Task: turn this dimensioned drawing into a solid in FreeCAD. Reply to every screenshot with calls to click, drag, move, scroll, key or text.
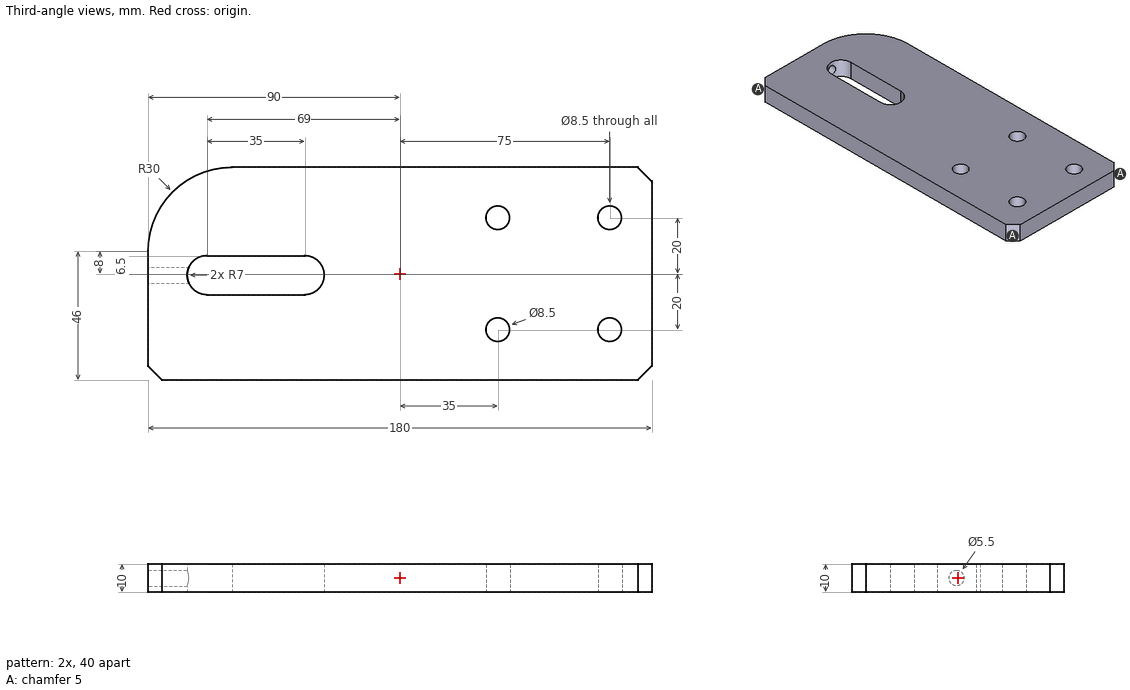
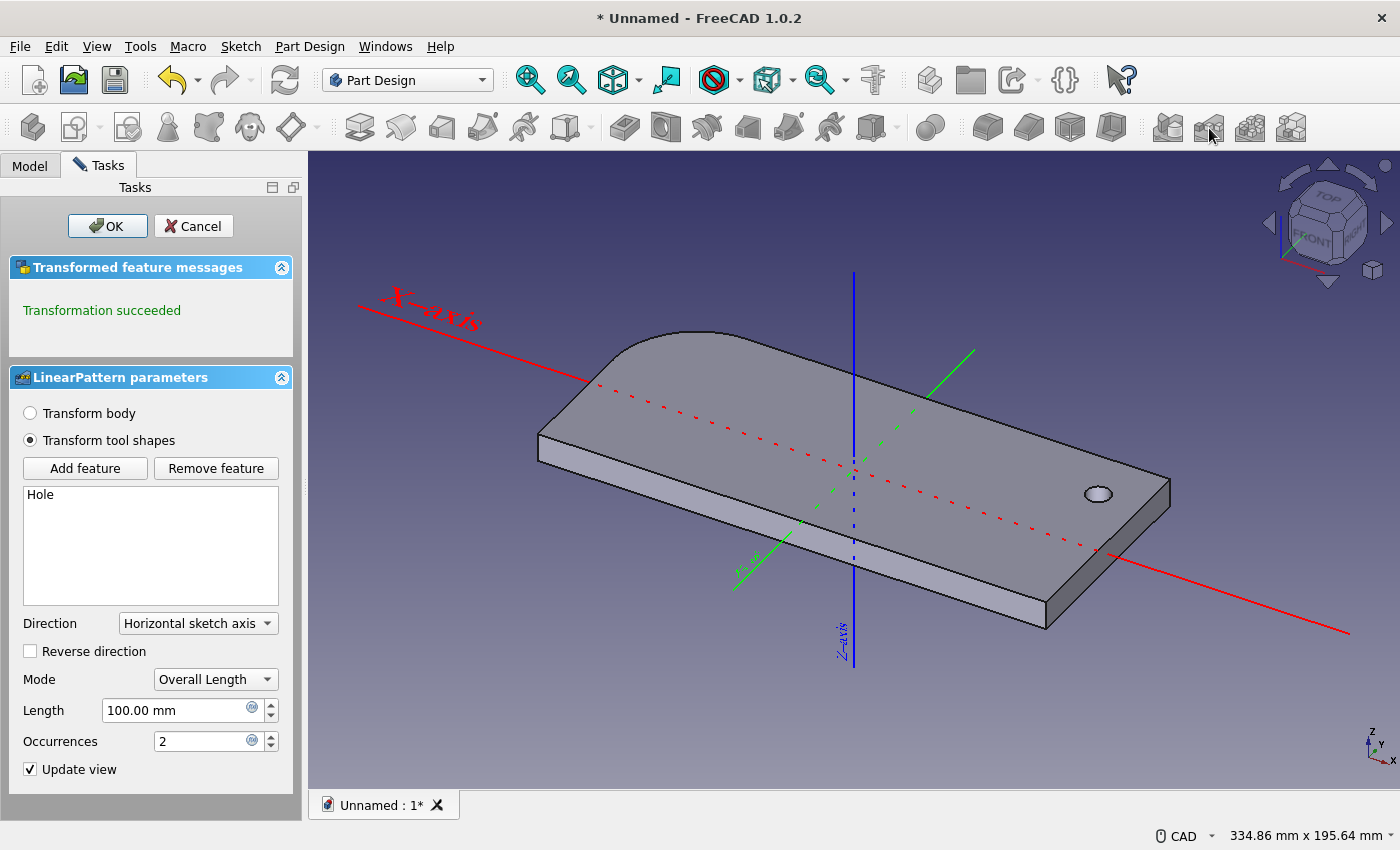
click(199, 624)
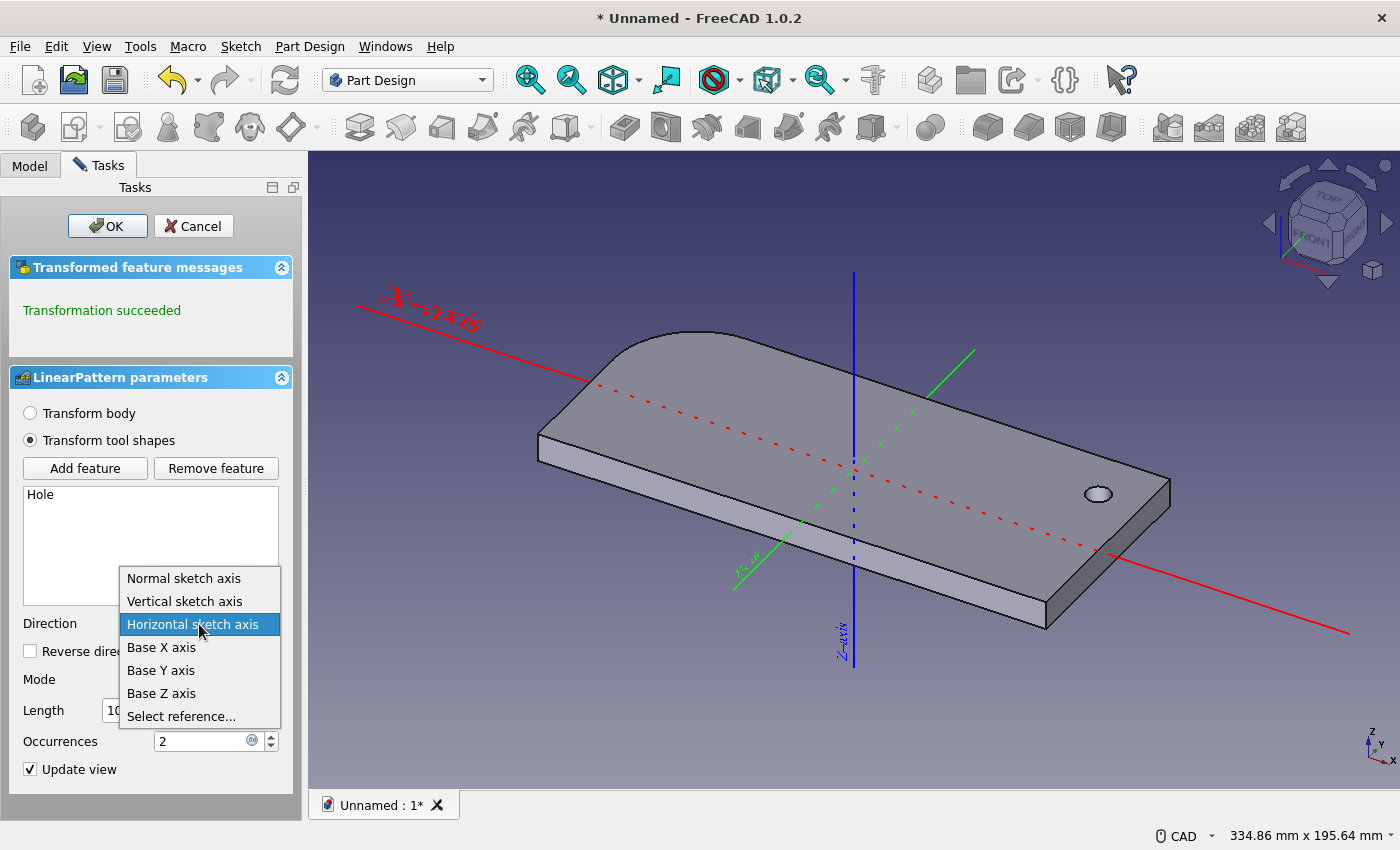
click(198, 648)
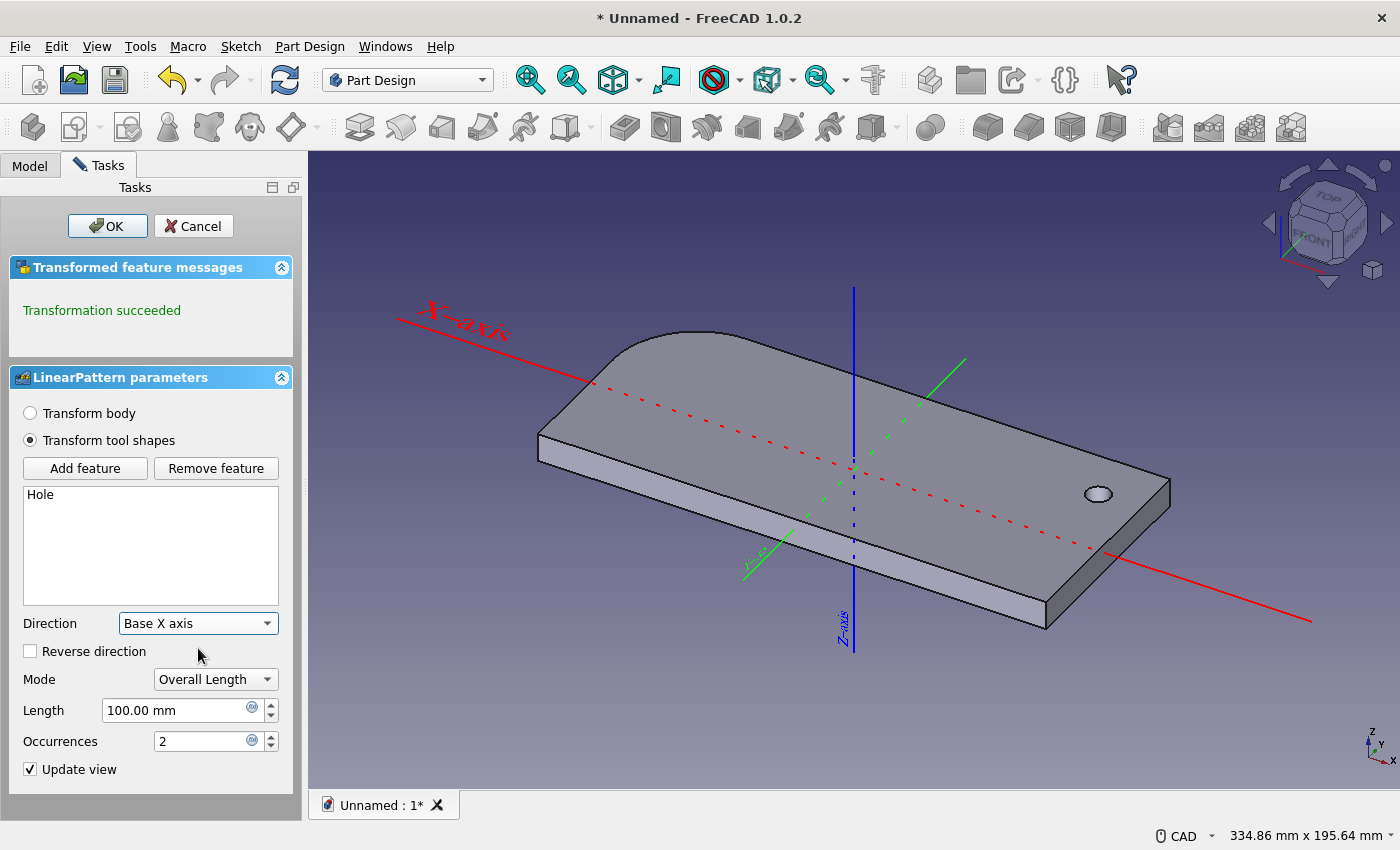
click(216, 680)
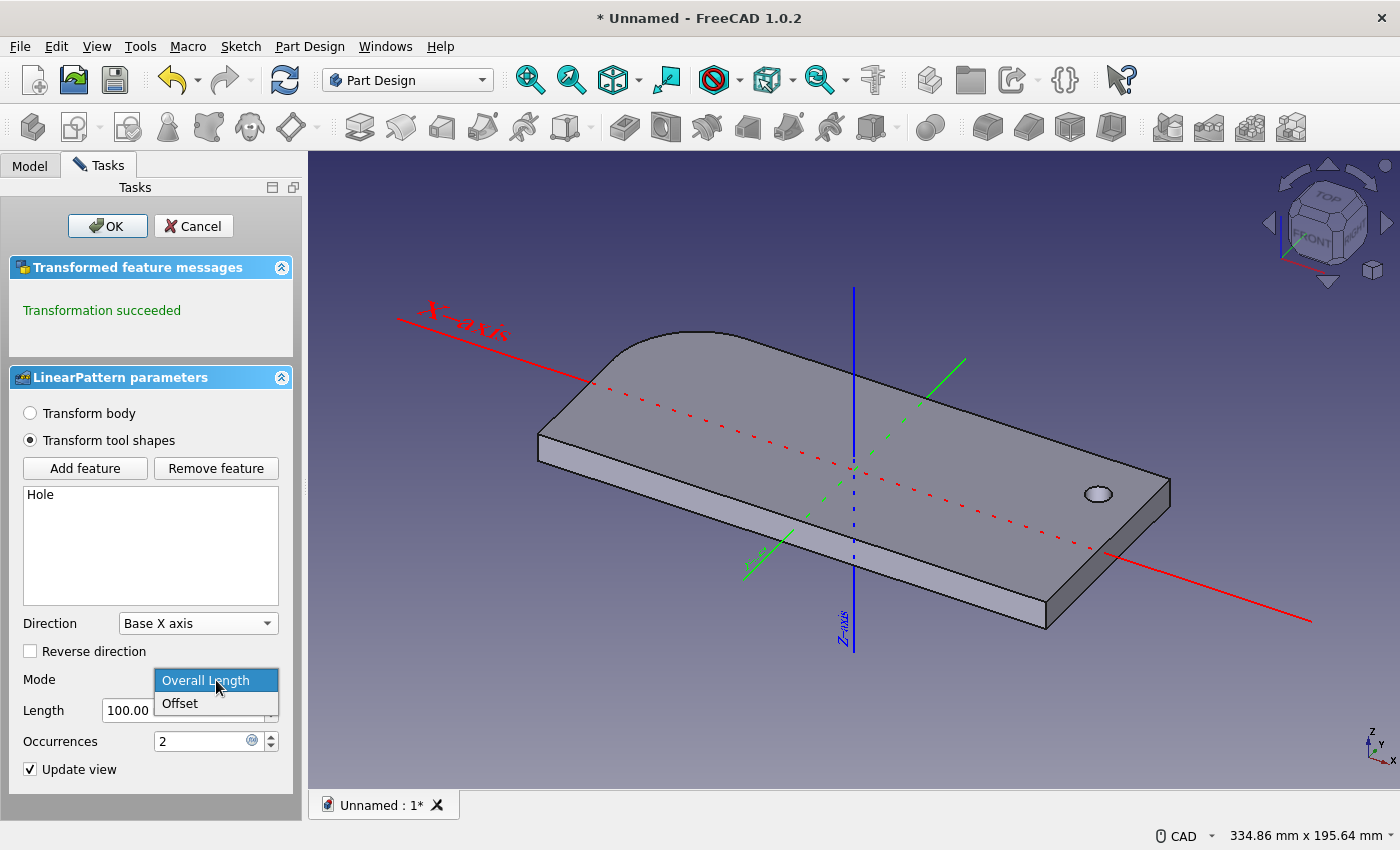
click(214, 704)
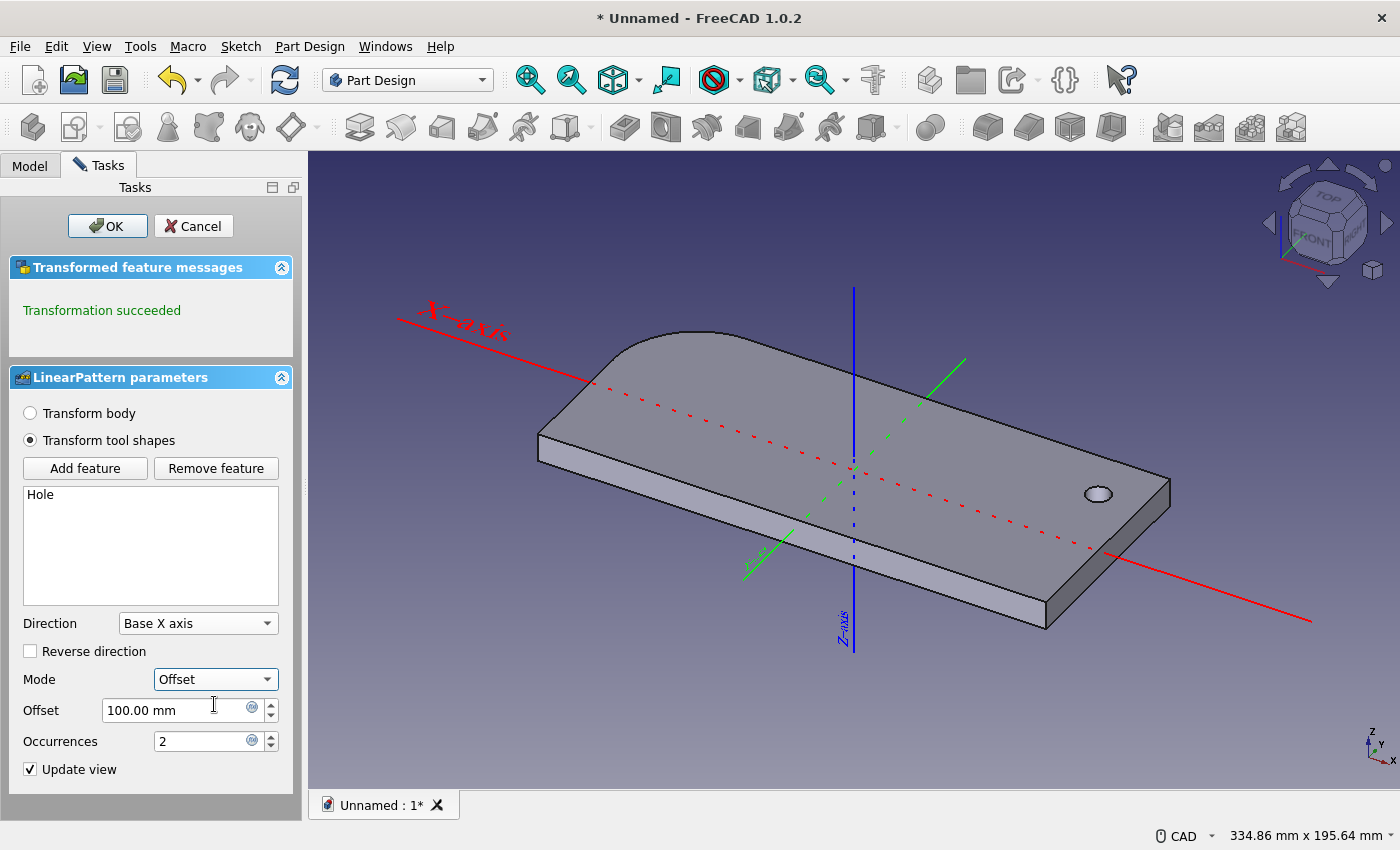
triple_click(184, 710)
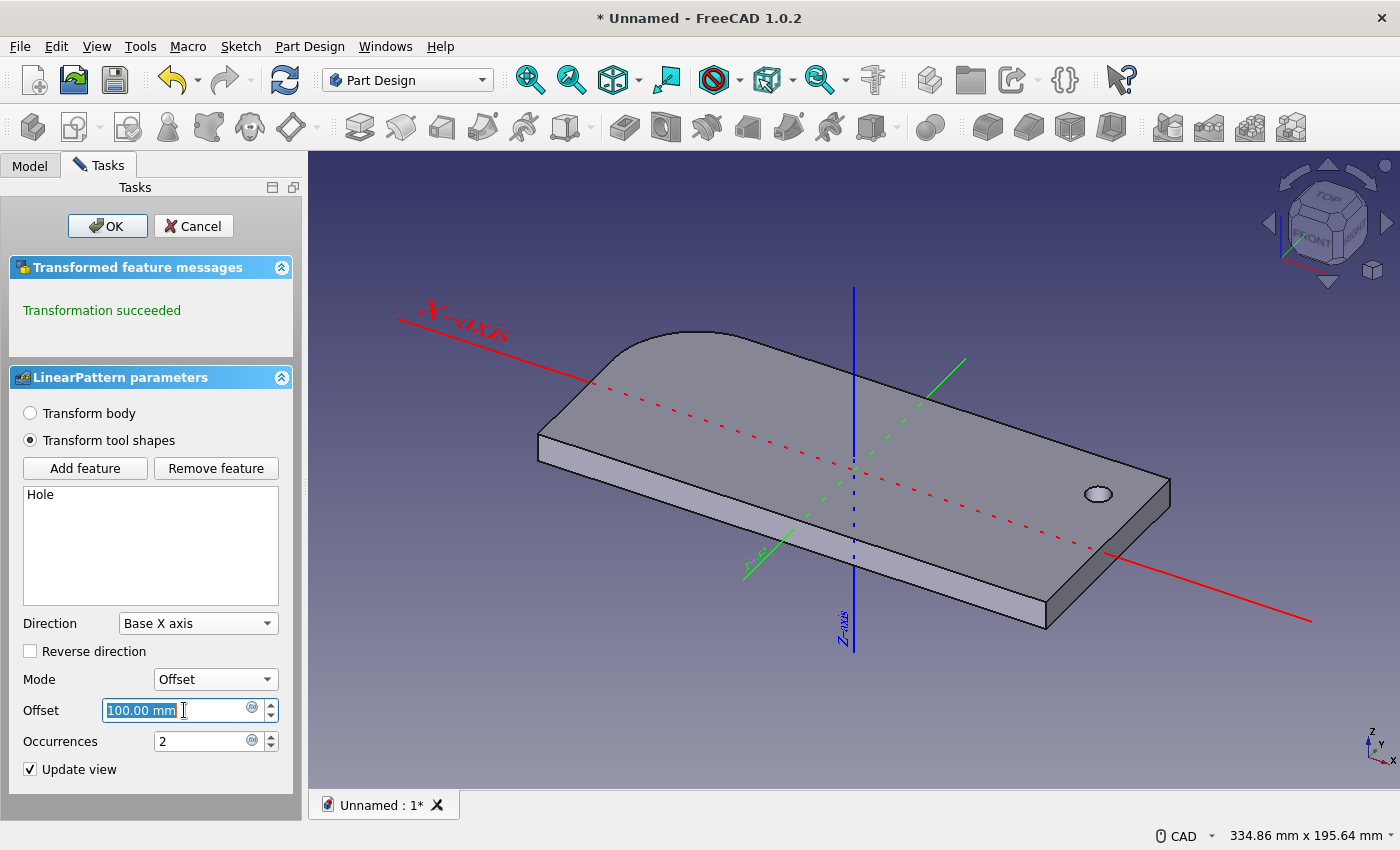
text(40)
key(Tab)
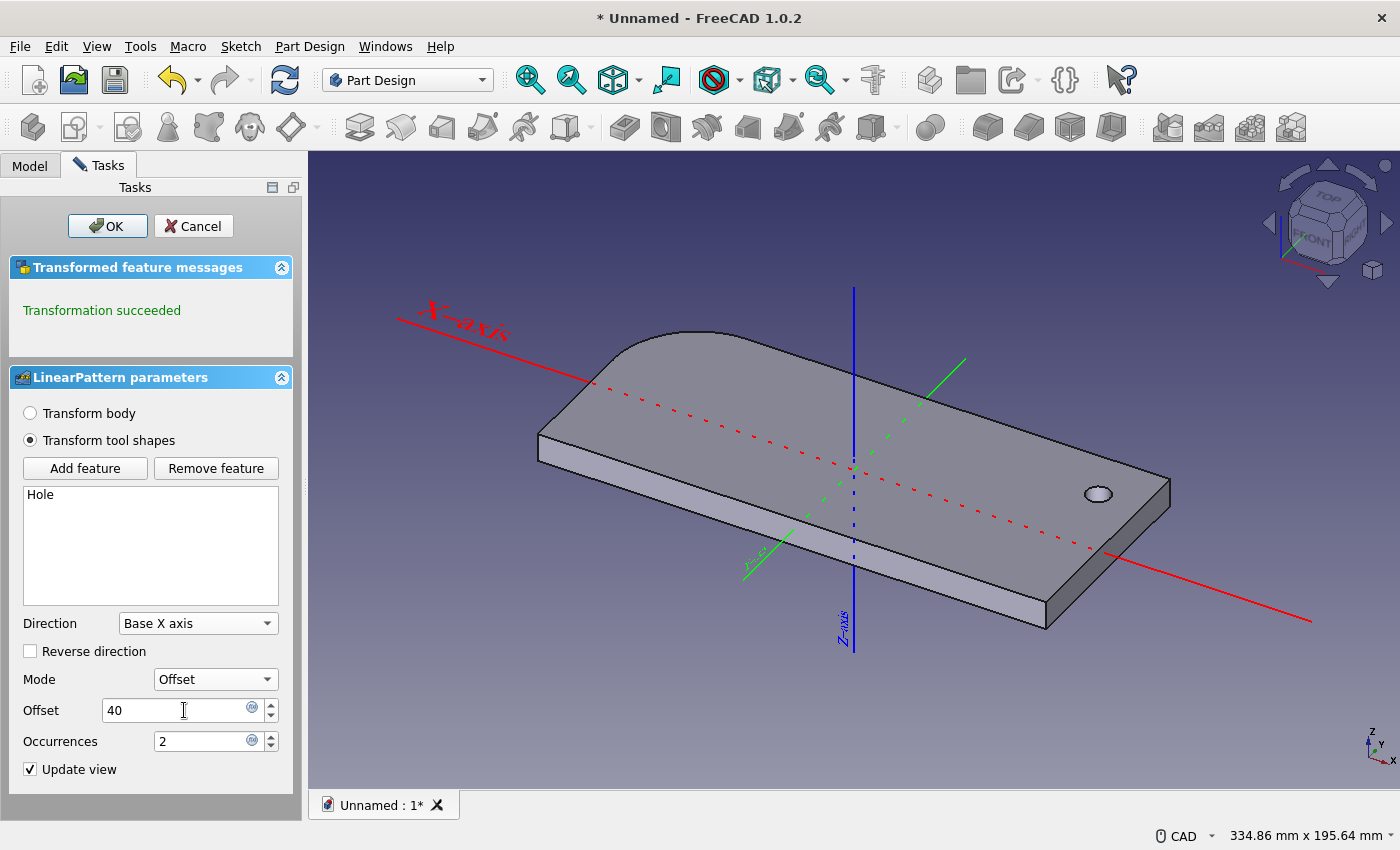
triple_click(210, 742)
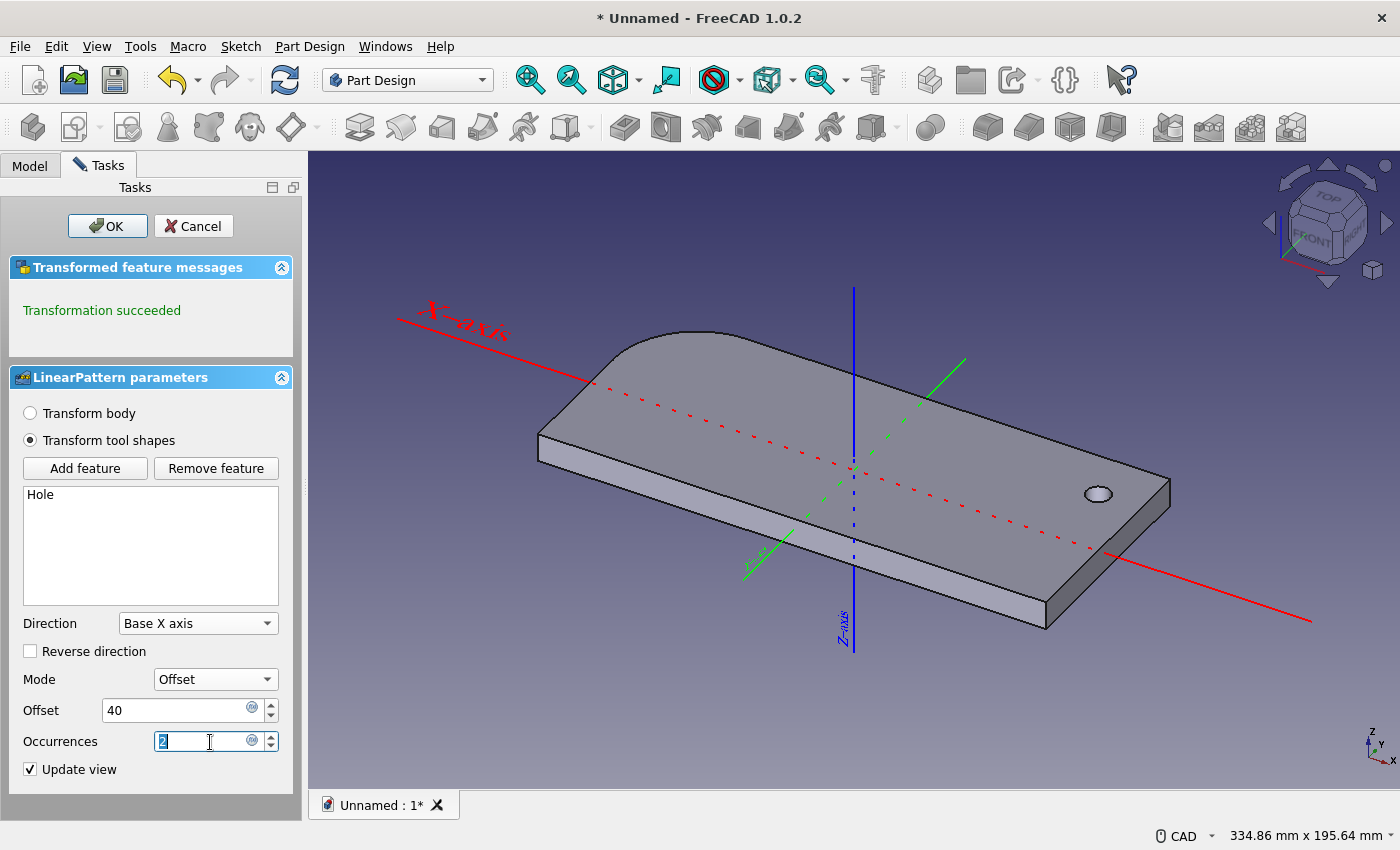
text(2)
key(Tab)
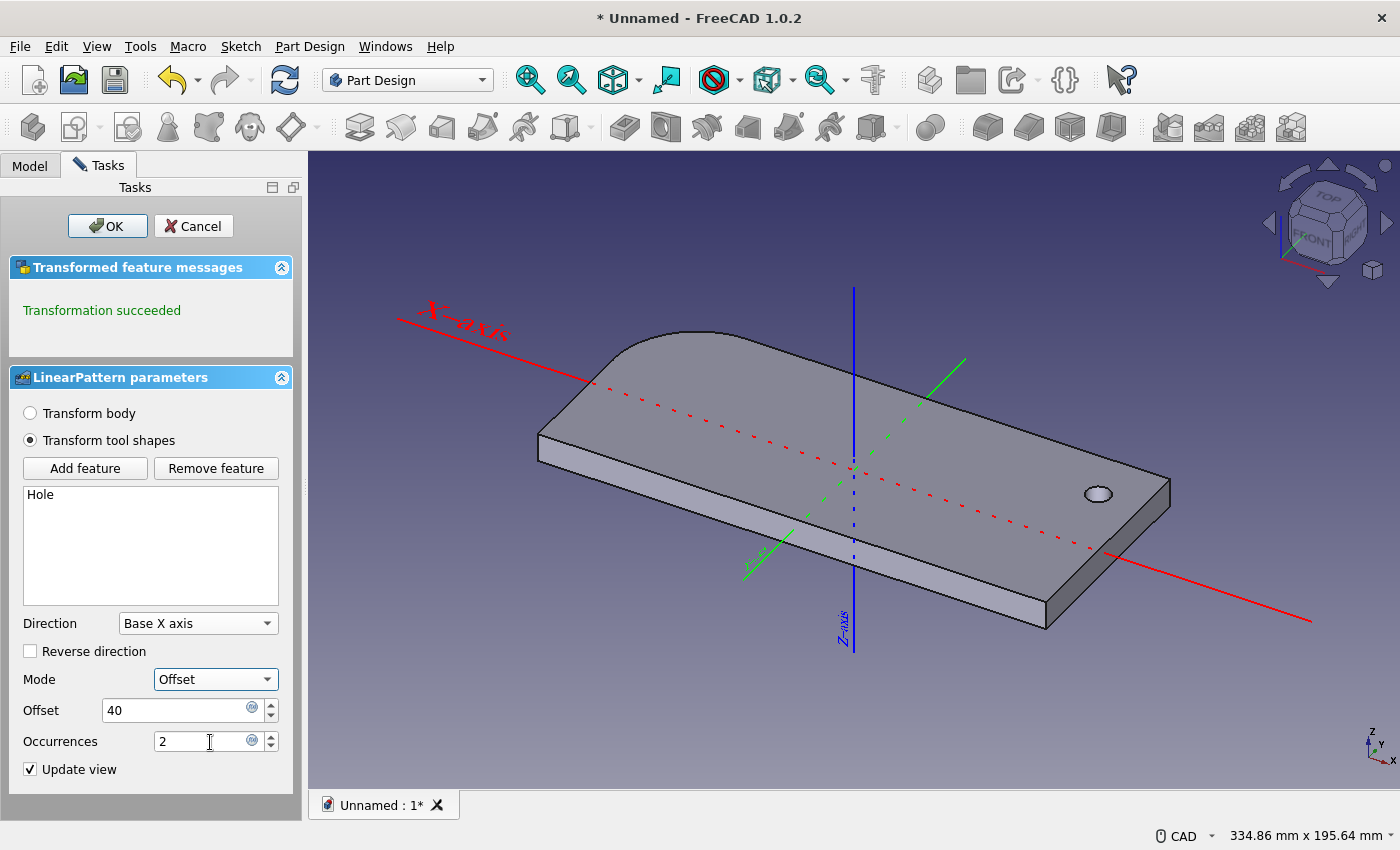
click(31, 651)